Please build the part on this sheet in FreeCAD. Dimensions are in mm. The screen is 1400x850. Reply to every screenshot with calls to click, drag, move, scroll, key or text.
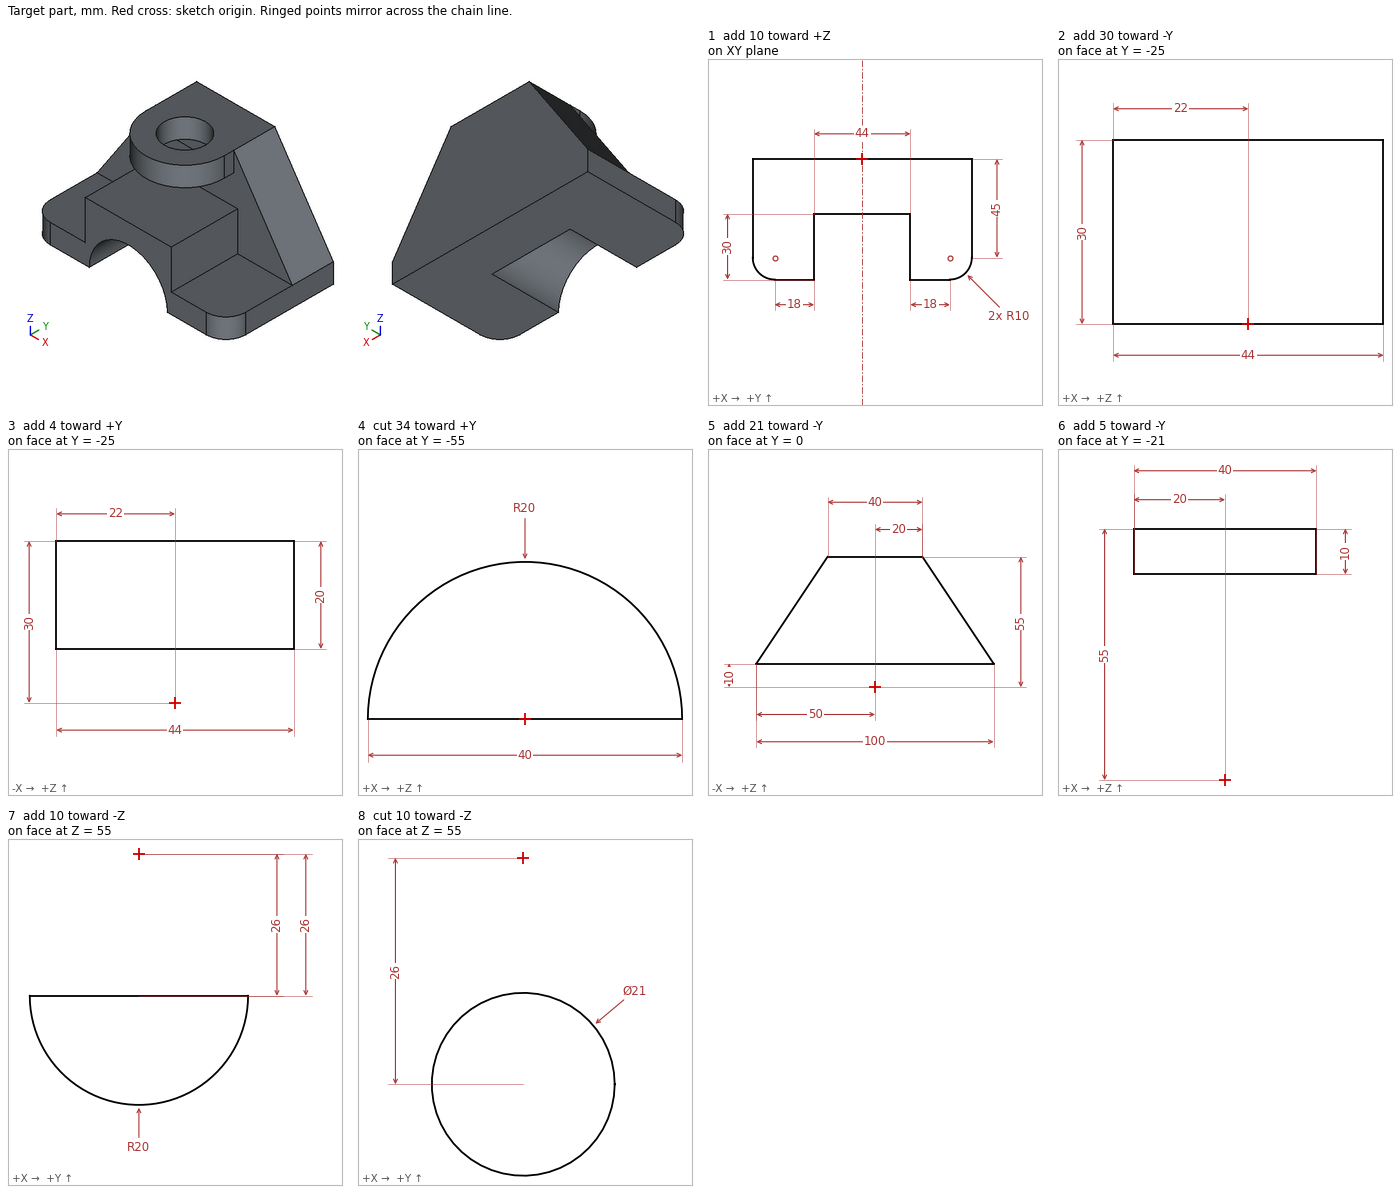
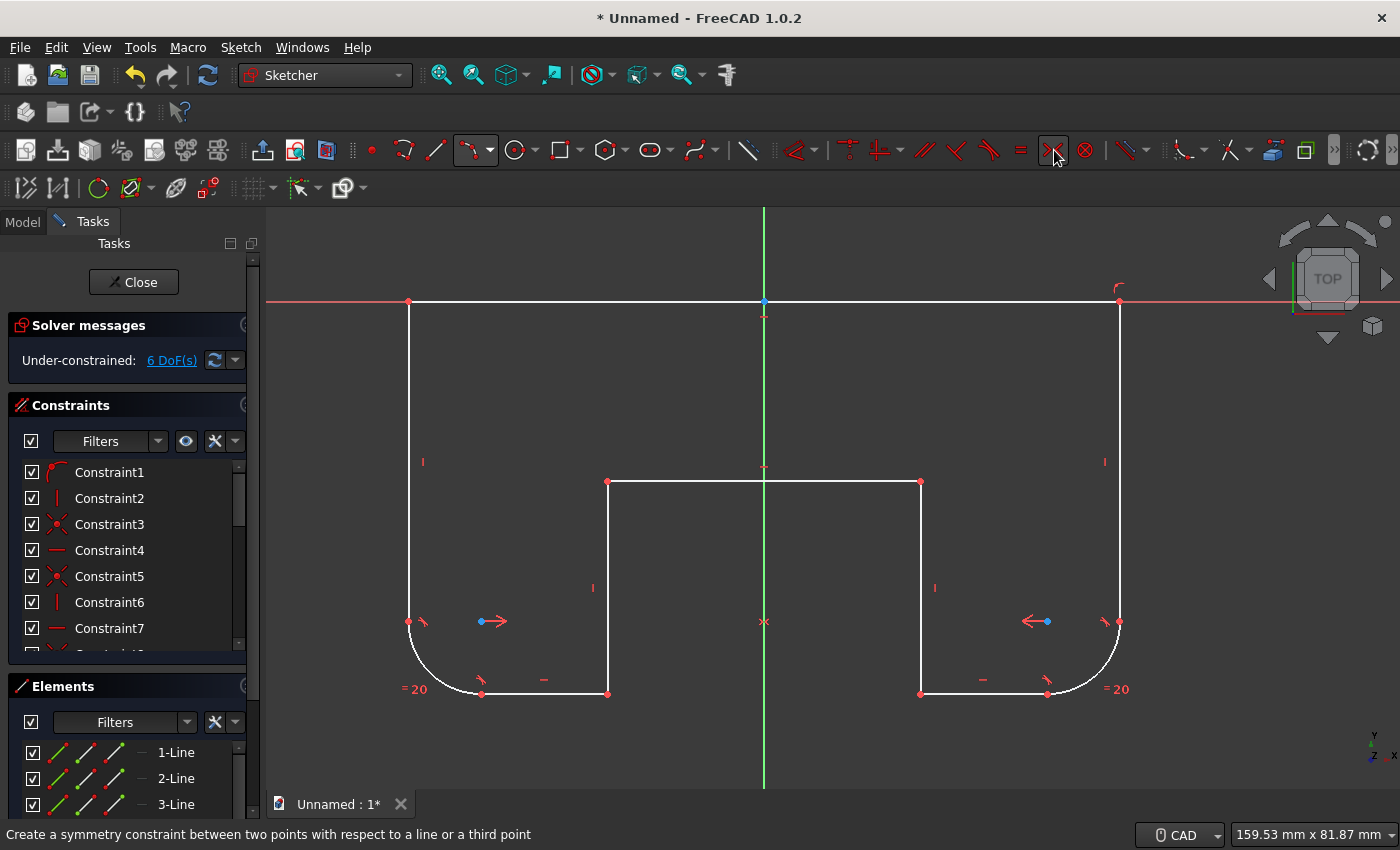
click(417, 654)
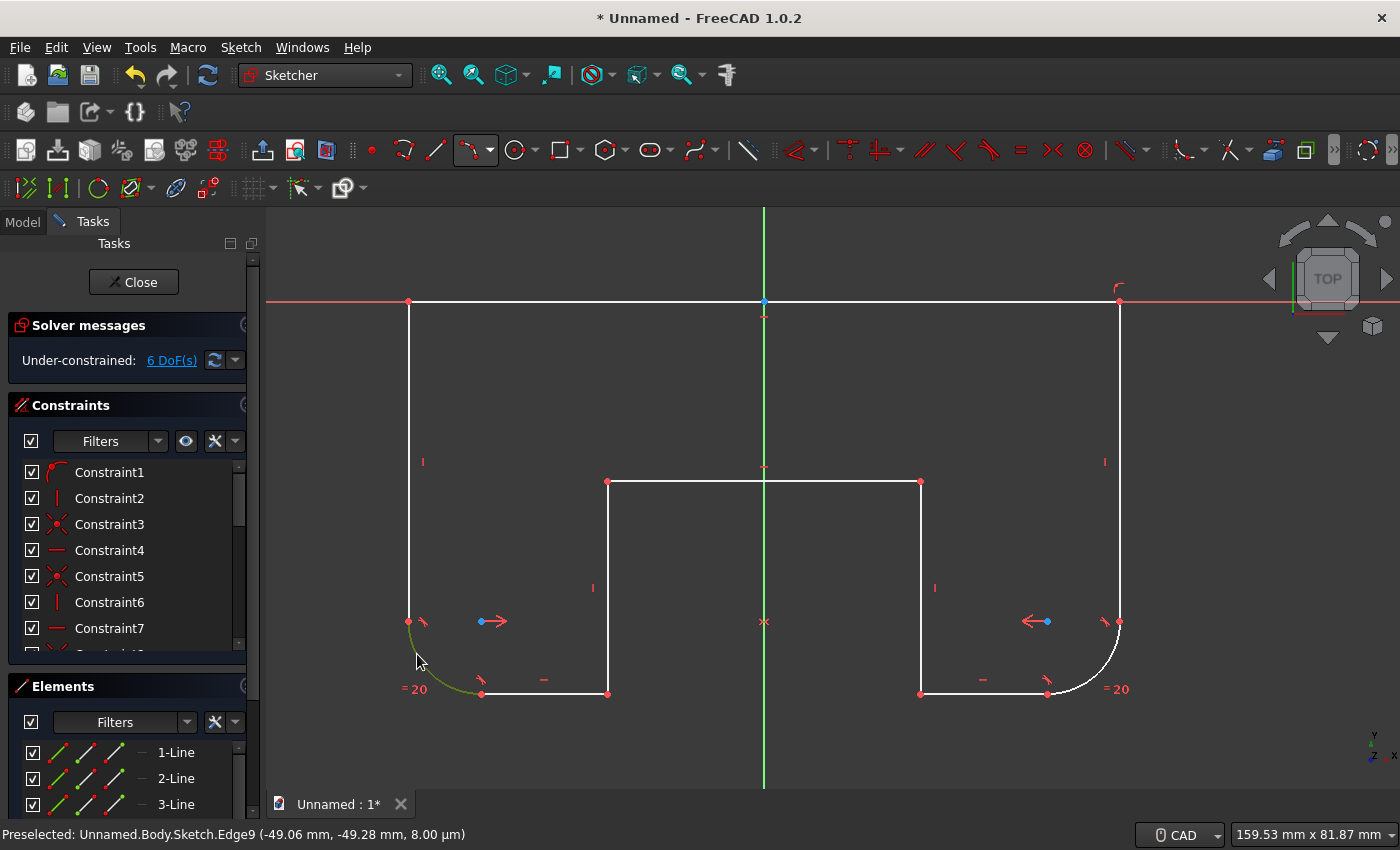
key(k)
key(r)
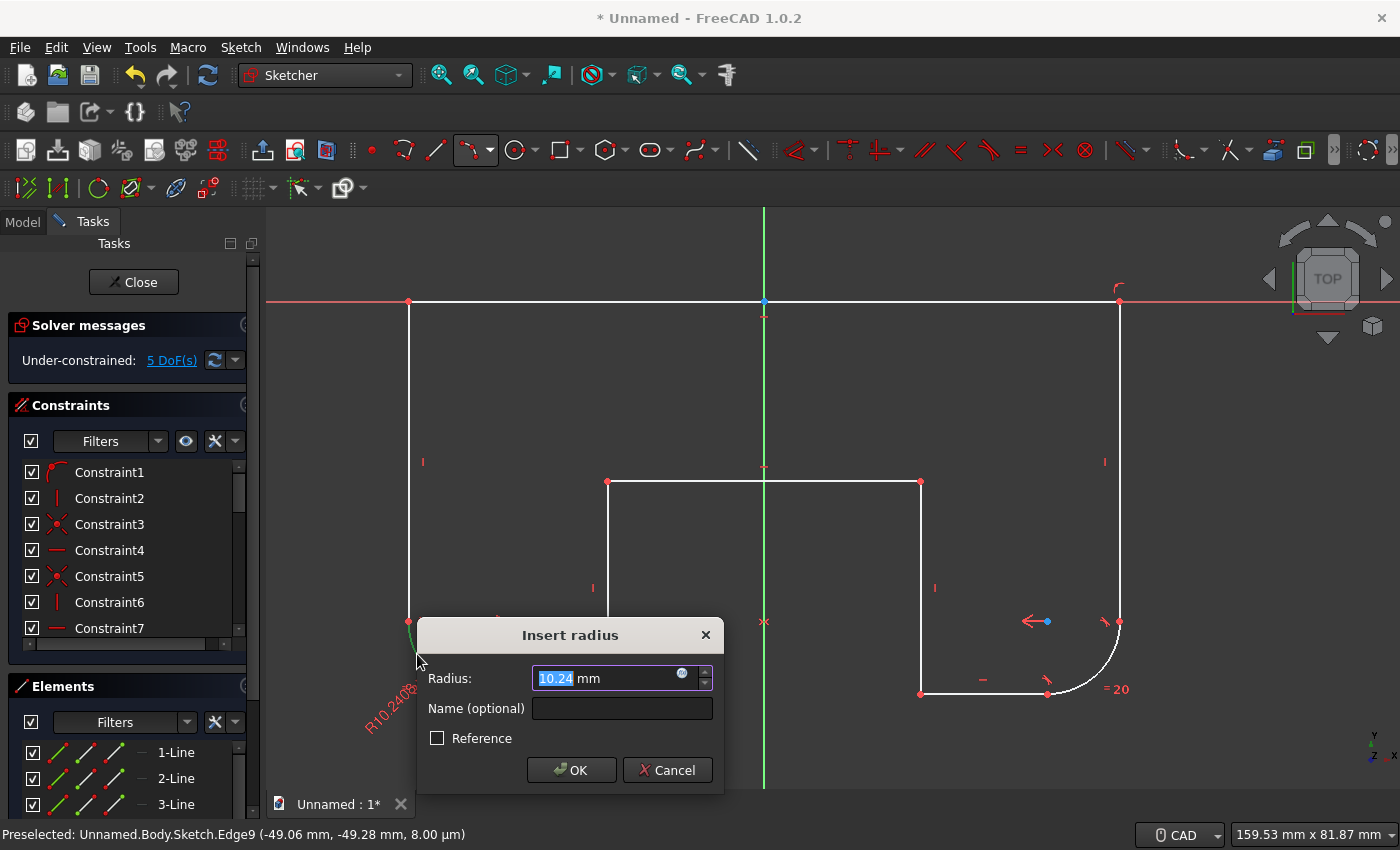
text(10)
key(Return)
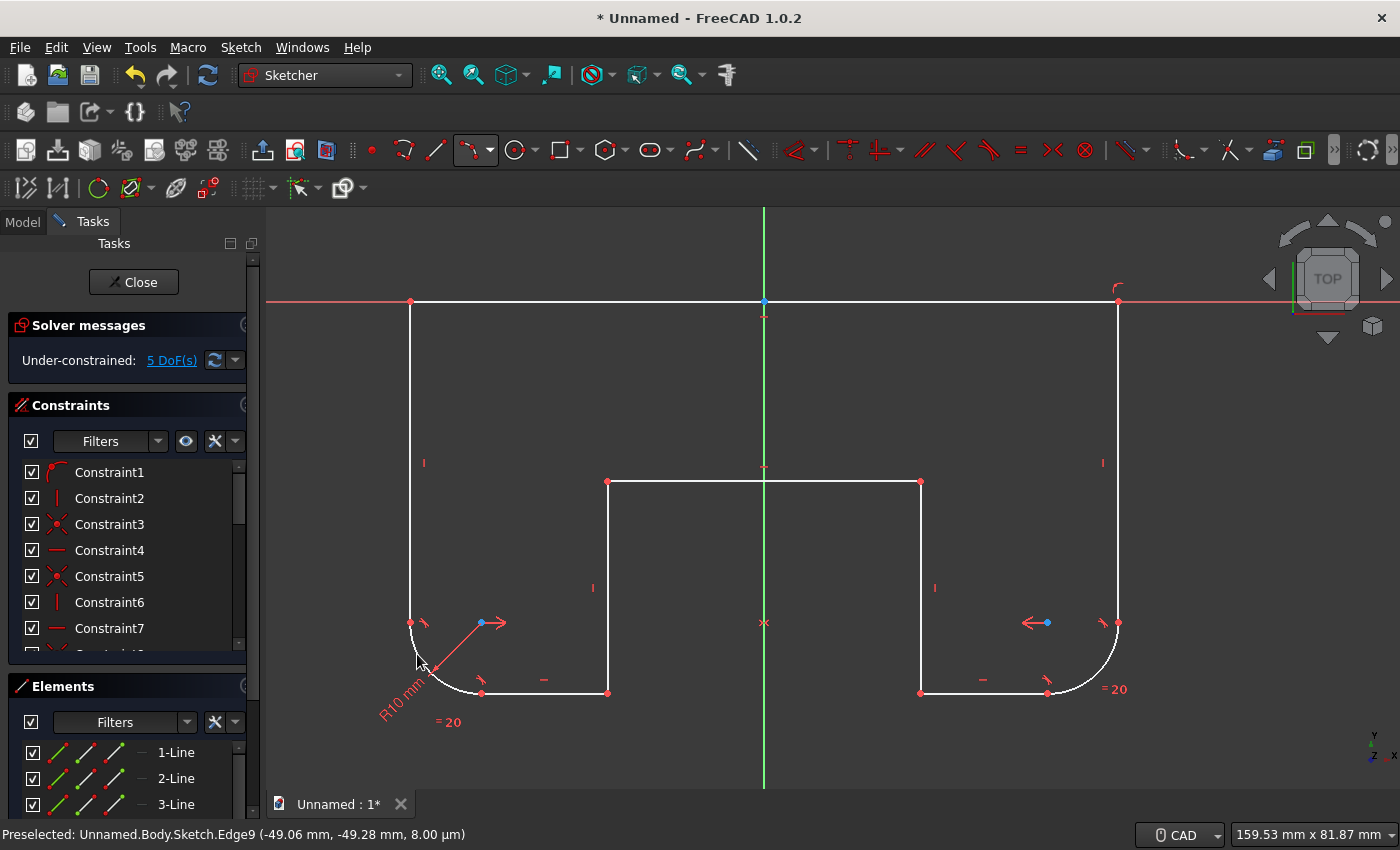
click(1118, 527)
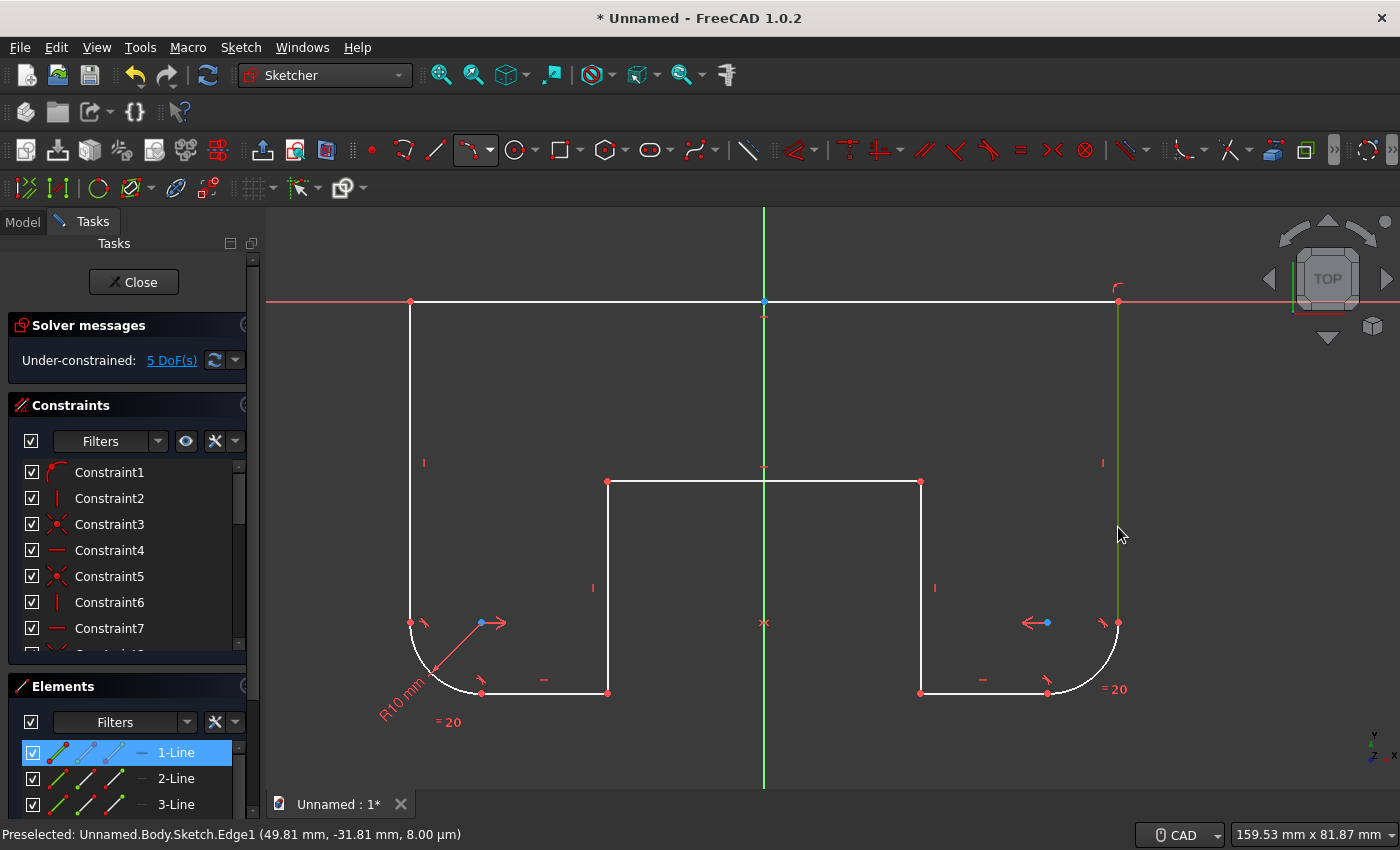
click(816, 150)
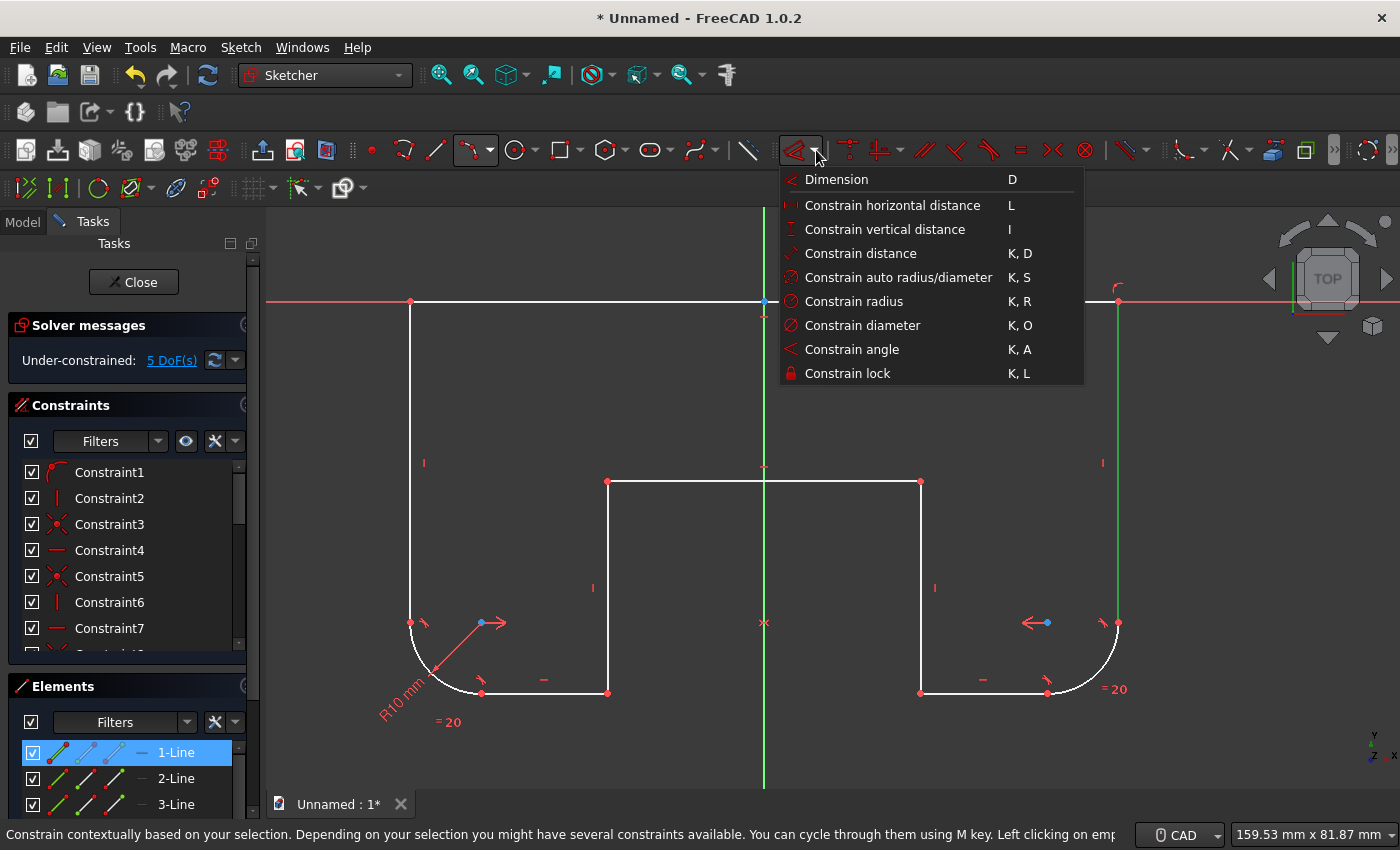
click(932, 229)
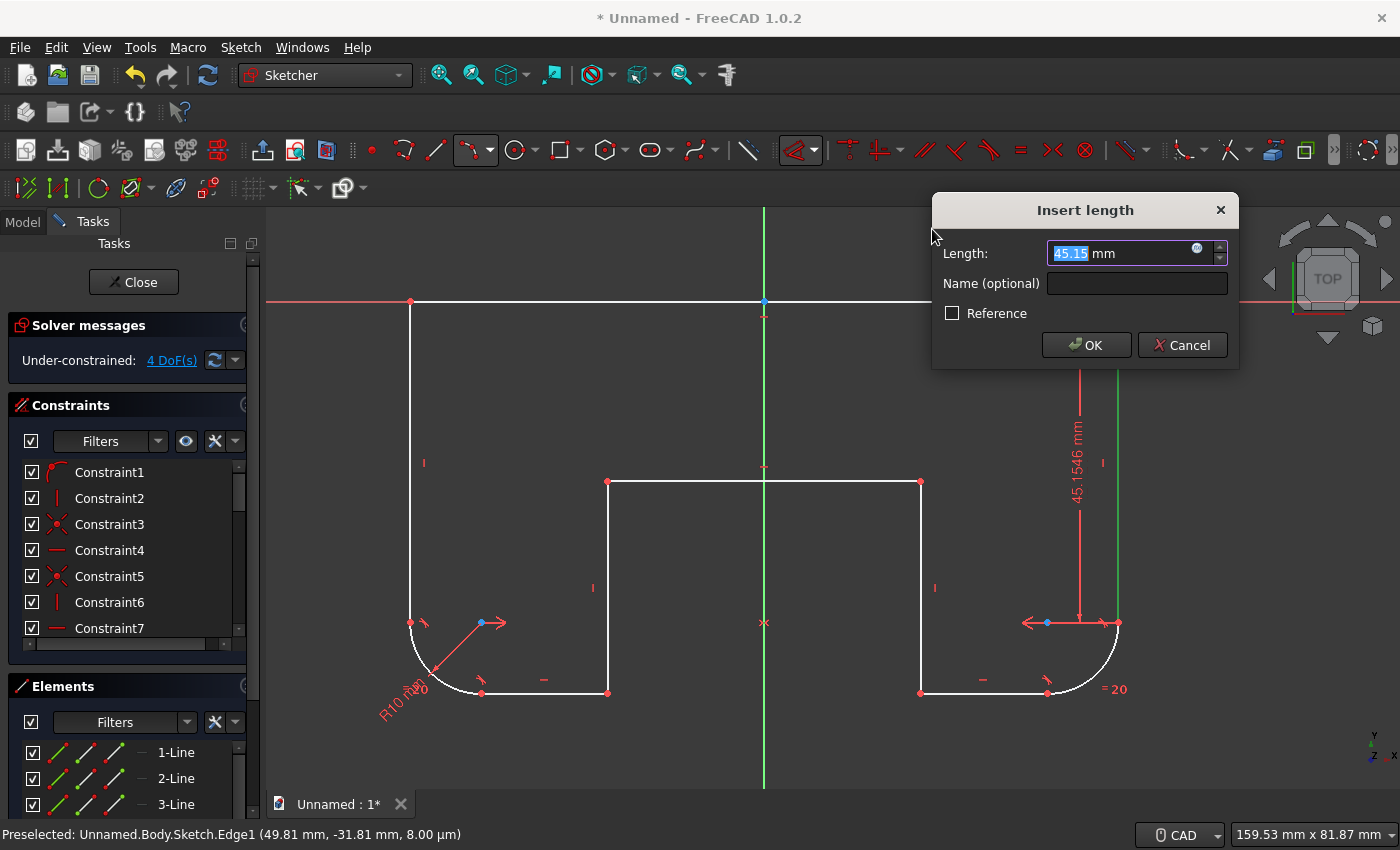
text(45)
key(Return)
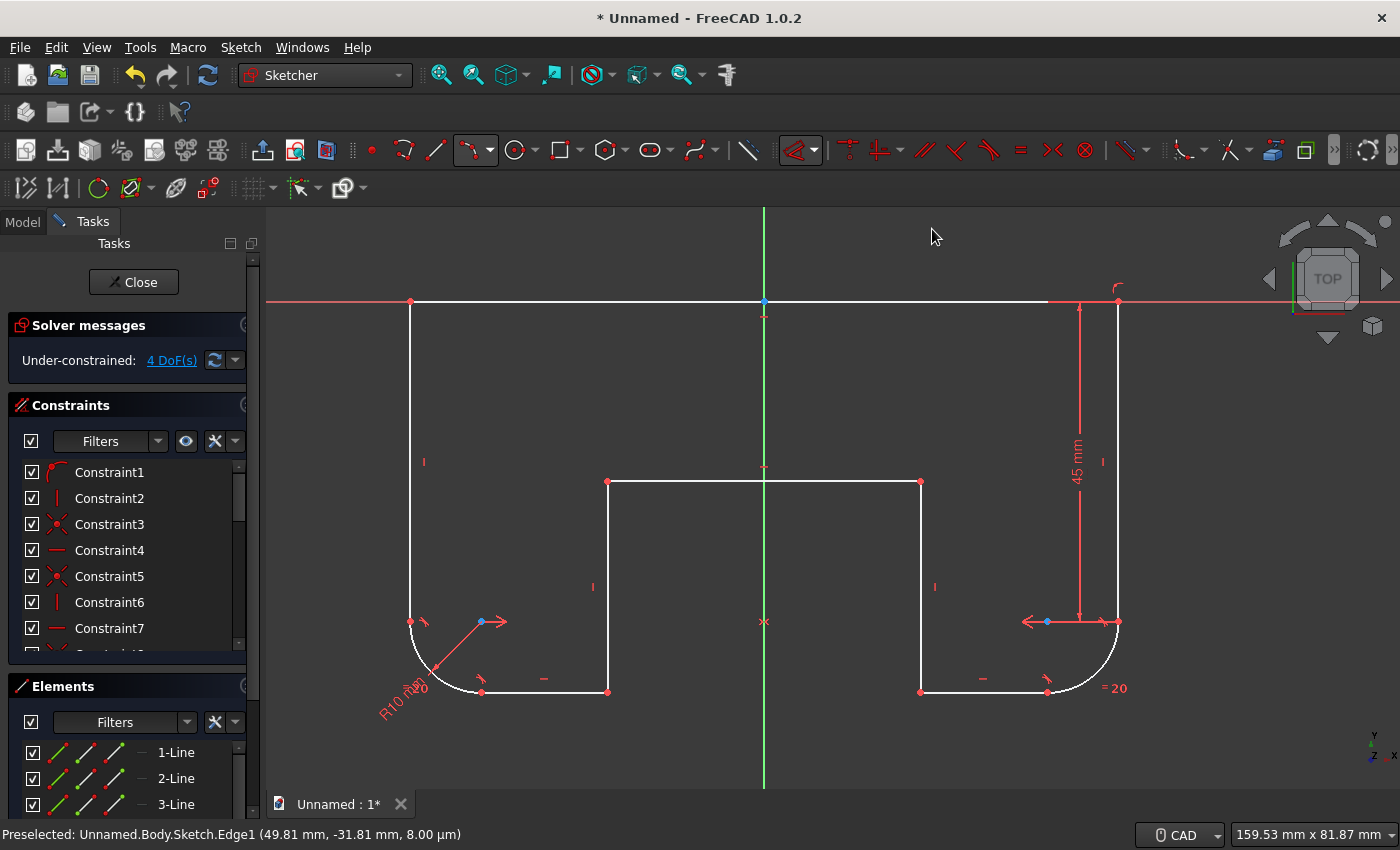
click(519, 693)